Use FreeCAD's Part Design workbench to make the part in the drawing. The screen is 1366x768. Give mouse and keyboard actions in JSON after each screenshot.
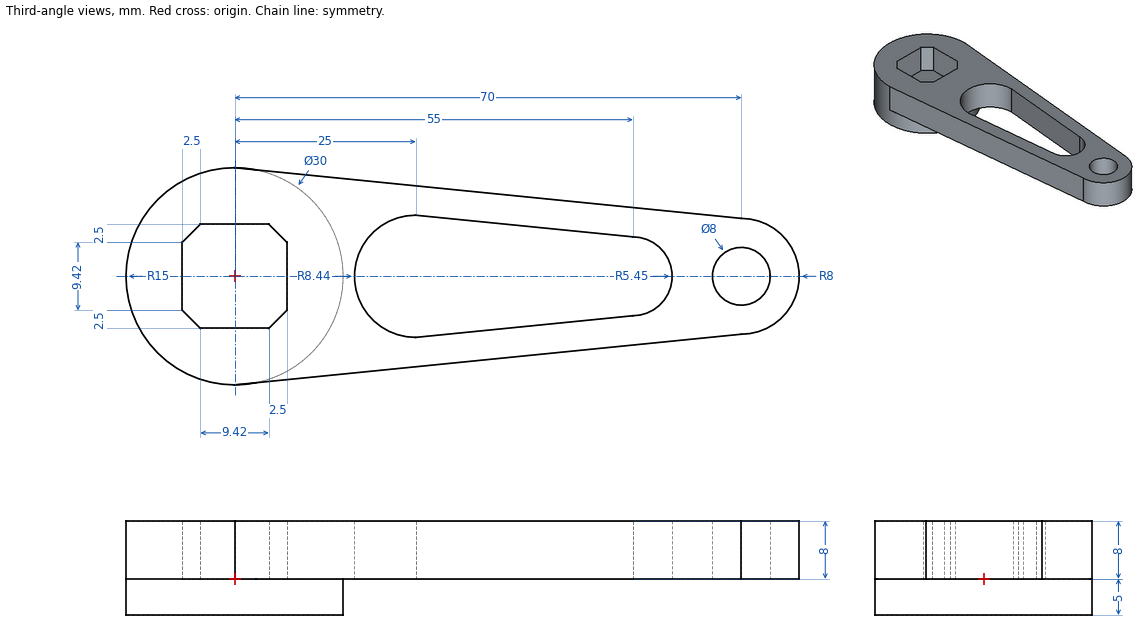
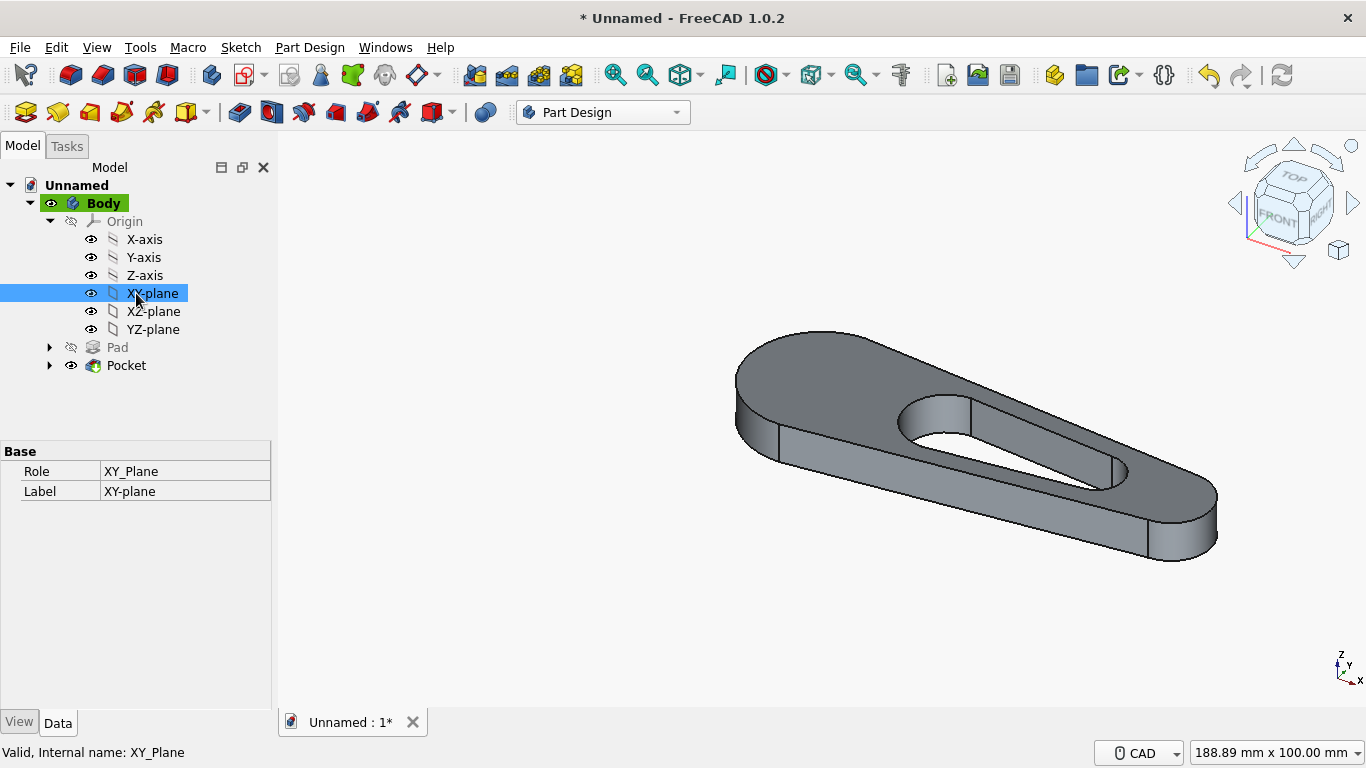
{"action": "left_click", "coordinate": [418, 76]}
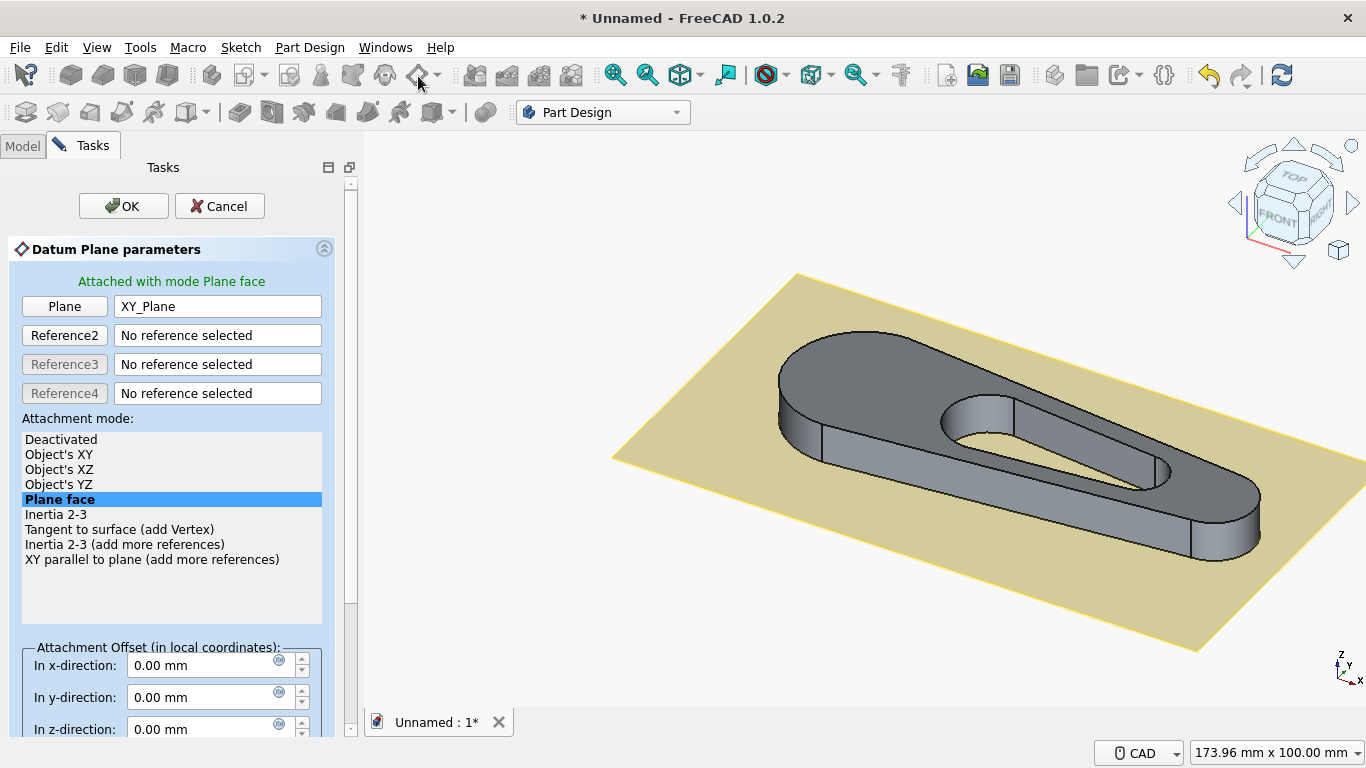
{"action": "scroll", "coordinate": [351, 456], "scroll_direction": "down", "scroll_amount": 2}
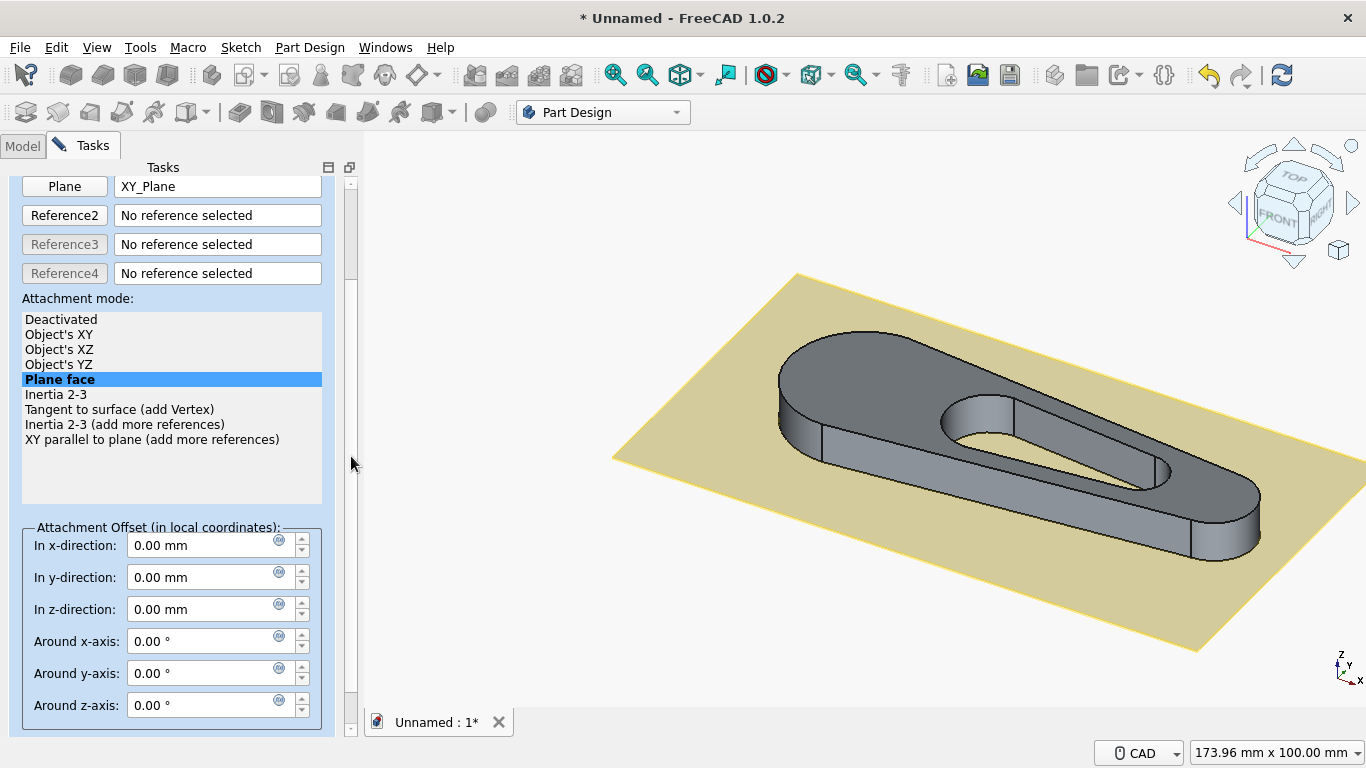
{"action": "triple_click", "coordinate": [210, 609]}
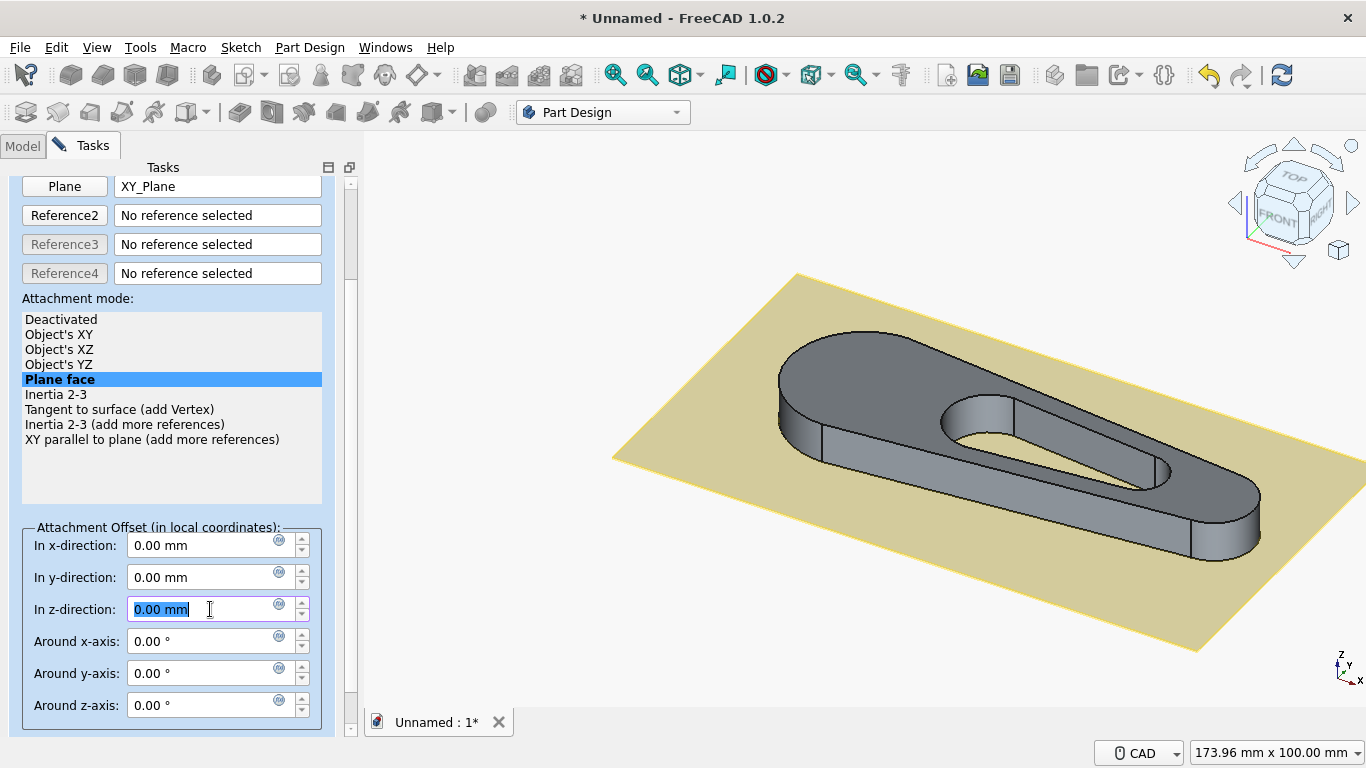
{"action": "type", "text": "-5"}
{"action": "key", "text": "Tab"}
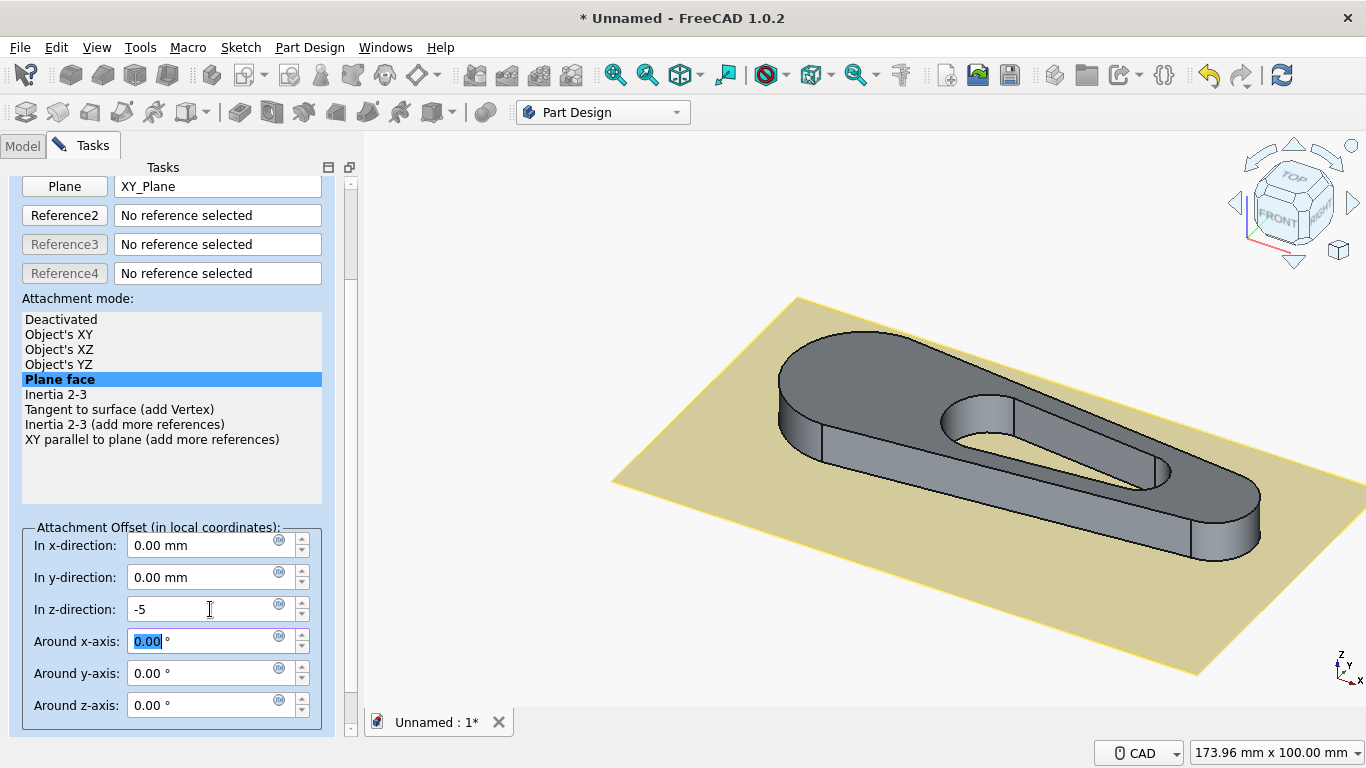
{"action": "scroll", "coordinate": [351, 456], "scroll_direction": "up", "scroll_amount": 3}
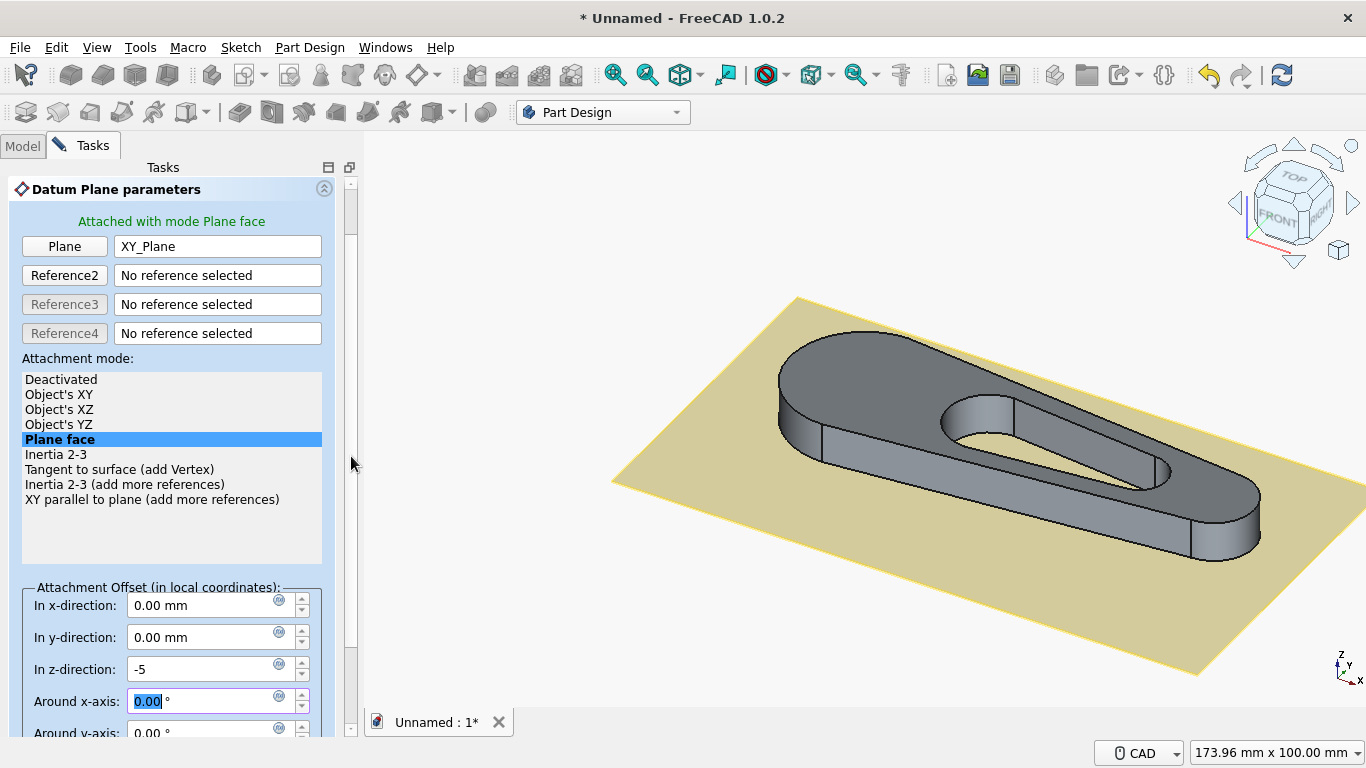
{"action": "left_click", "coordinate": [124, 206]}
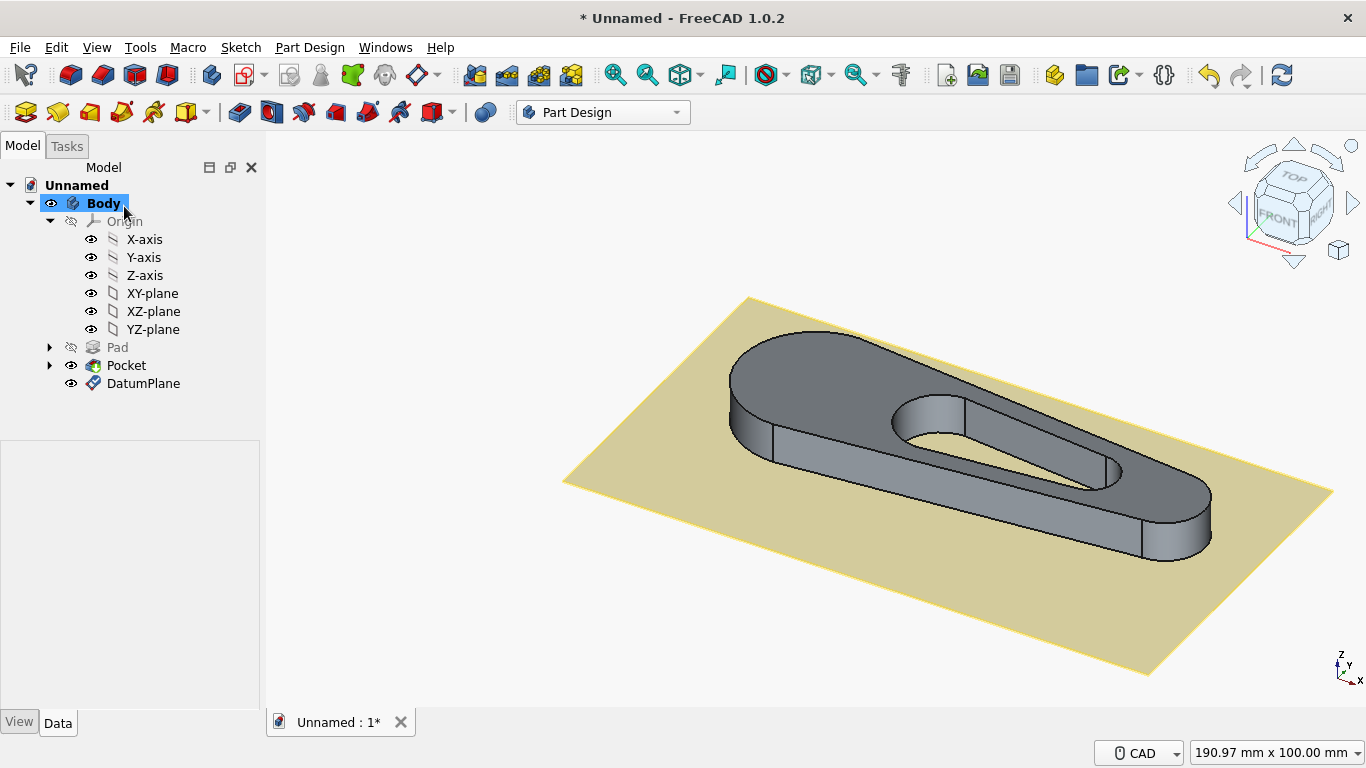
{"action": "left_click", "coordinate": [116, 383]}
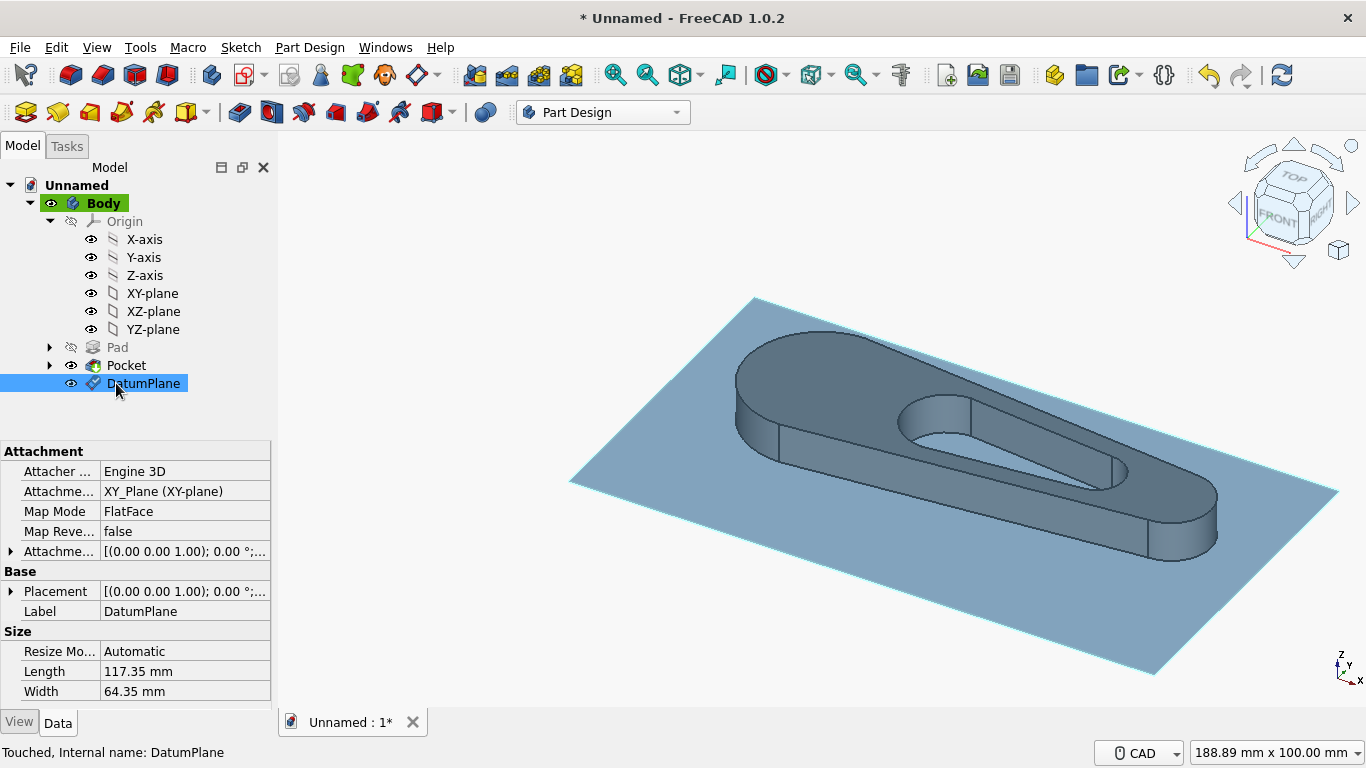
{"action": "left_click", "coordinate": [244, 76]}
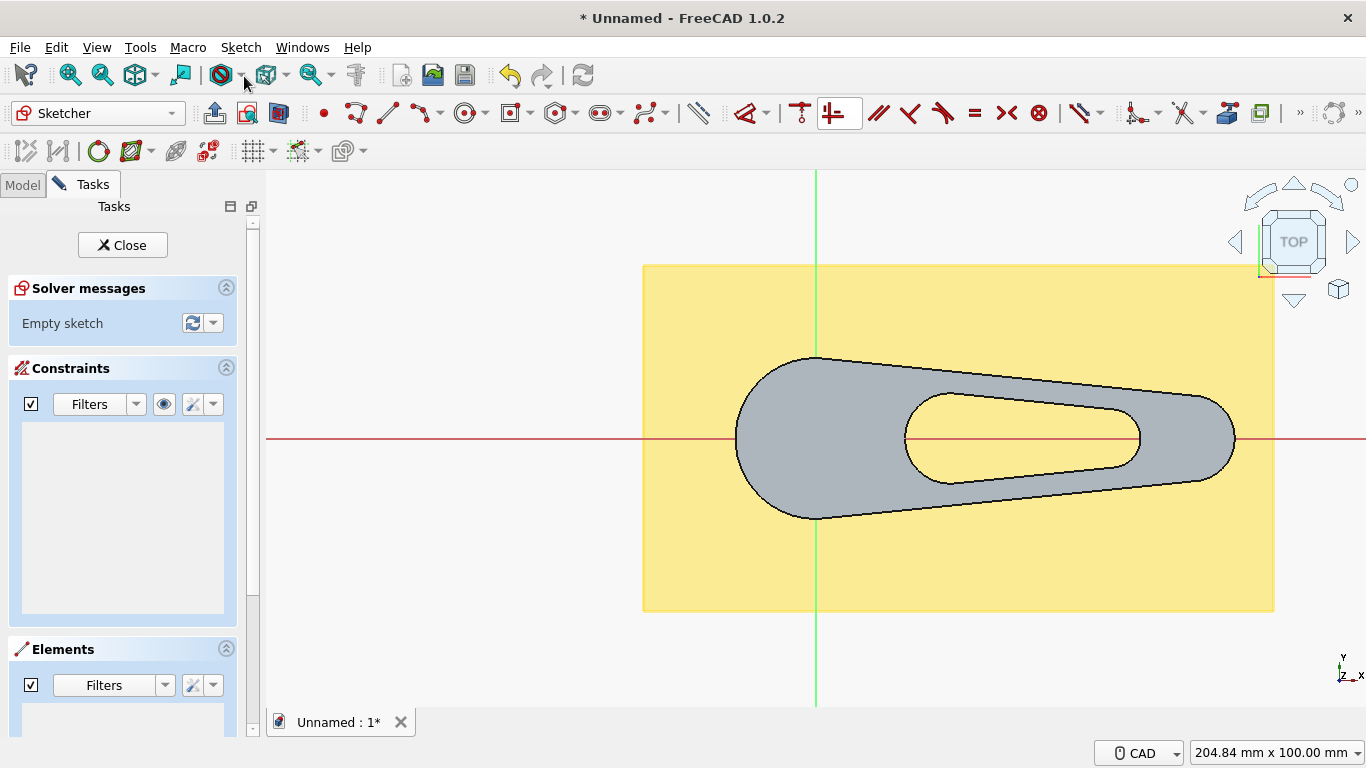
{"action": "left_click", "coordinate": [280, 114]}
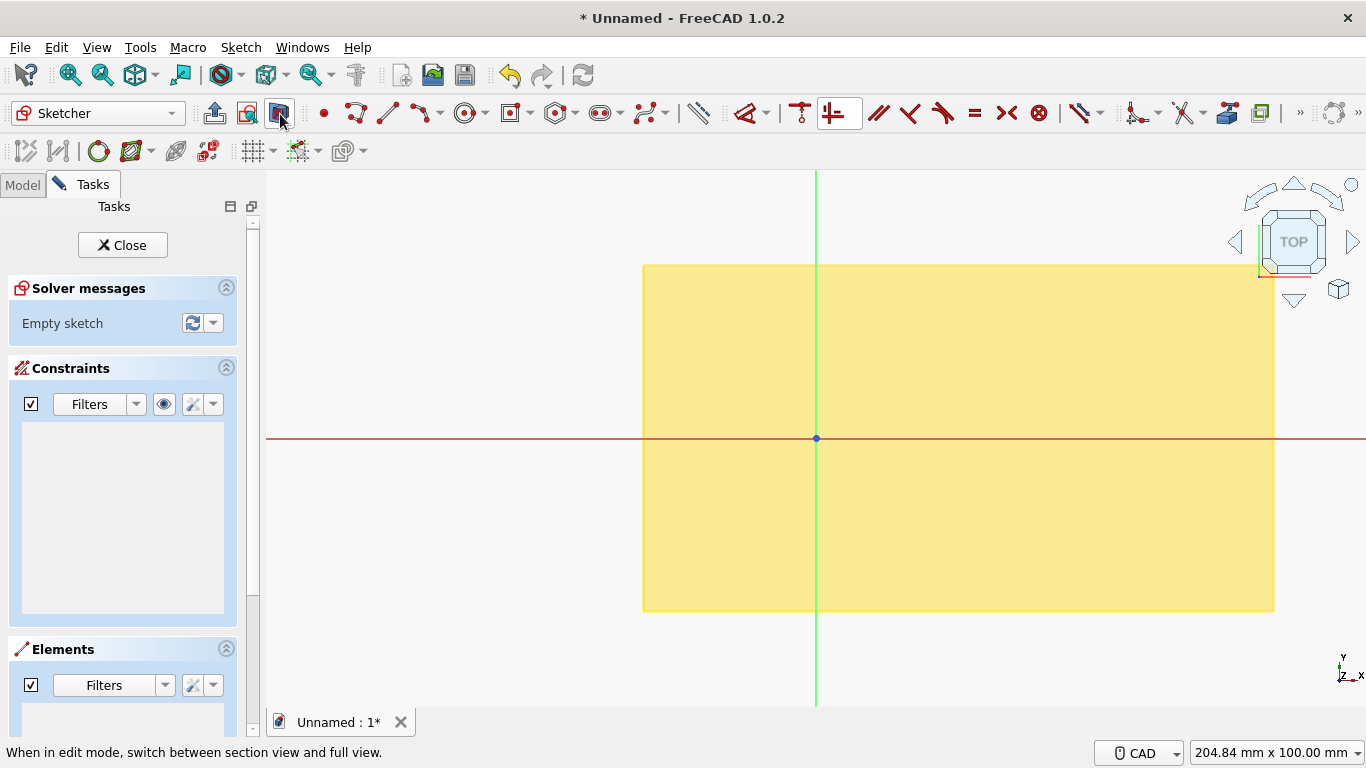
{"action": "scroll", "coordinate": [872, 438], "scroll_direction": "up", "scroll_amount": 4}